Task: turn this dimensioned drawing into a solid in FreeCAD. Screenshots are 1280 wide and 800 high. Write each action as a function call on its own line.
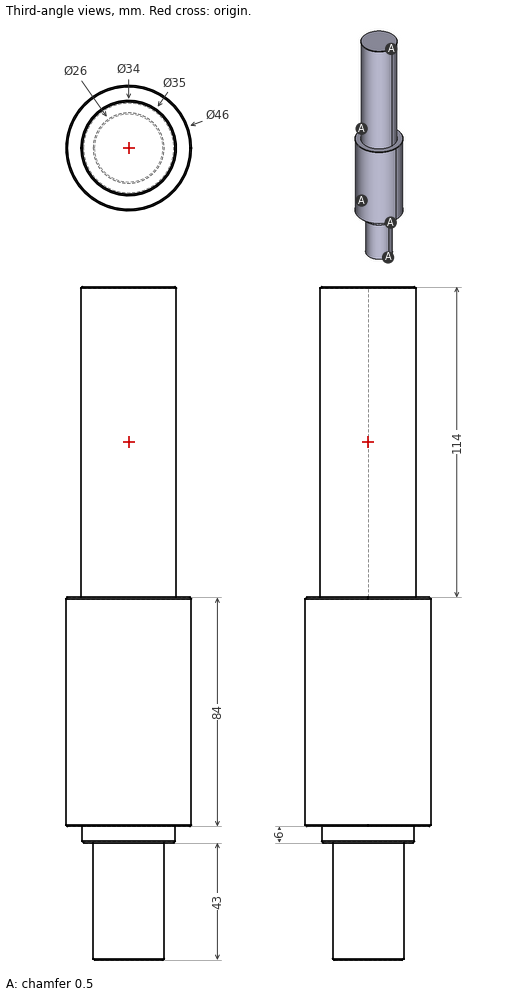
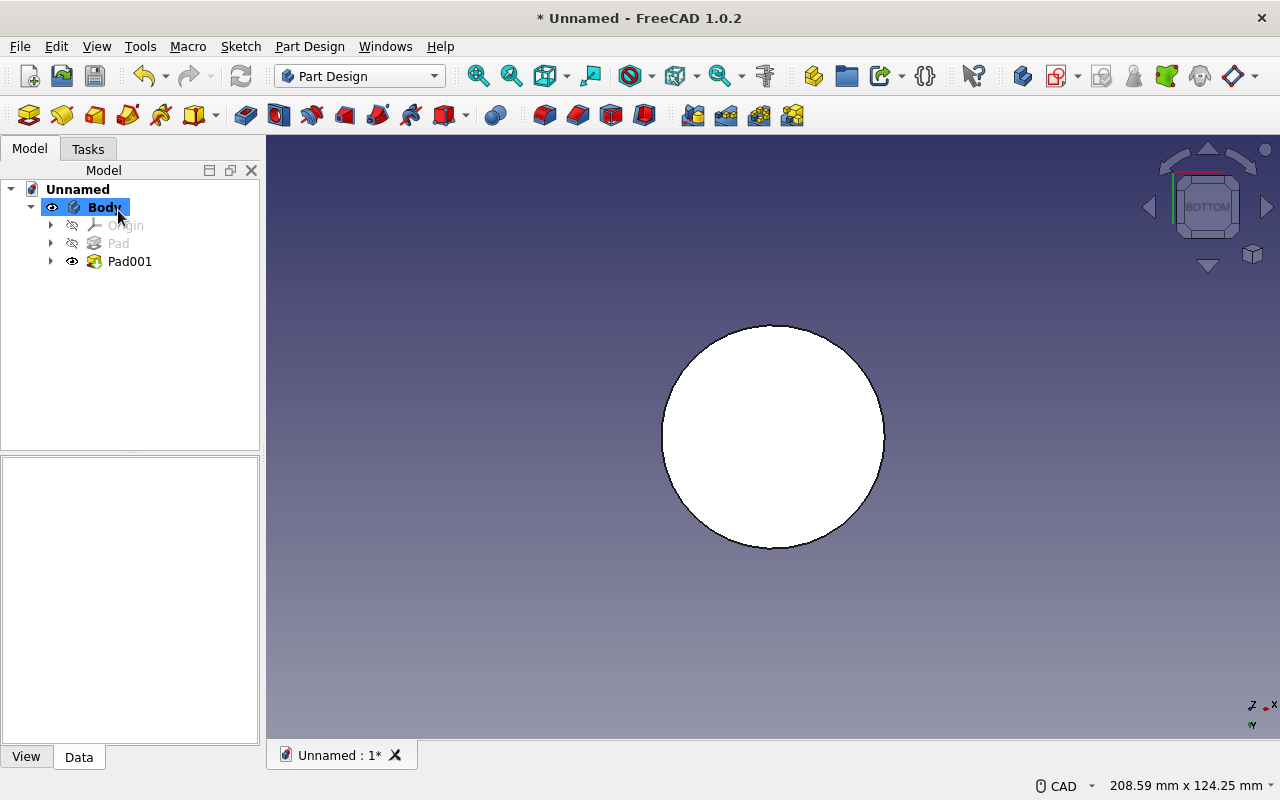
key(v)
key(f)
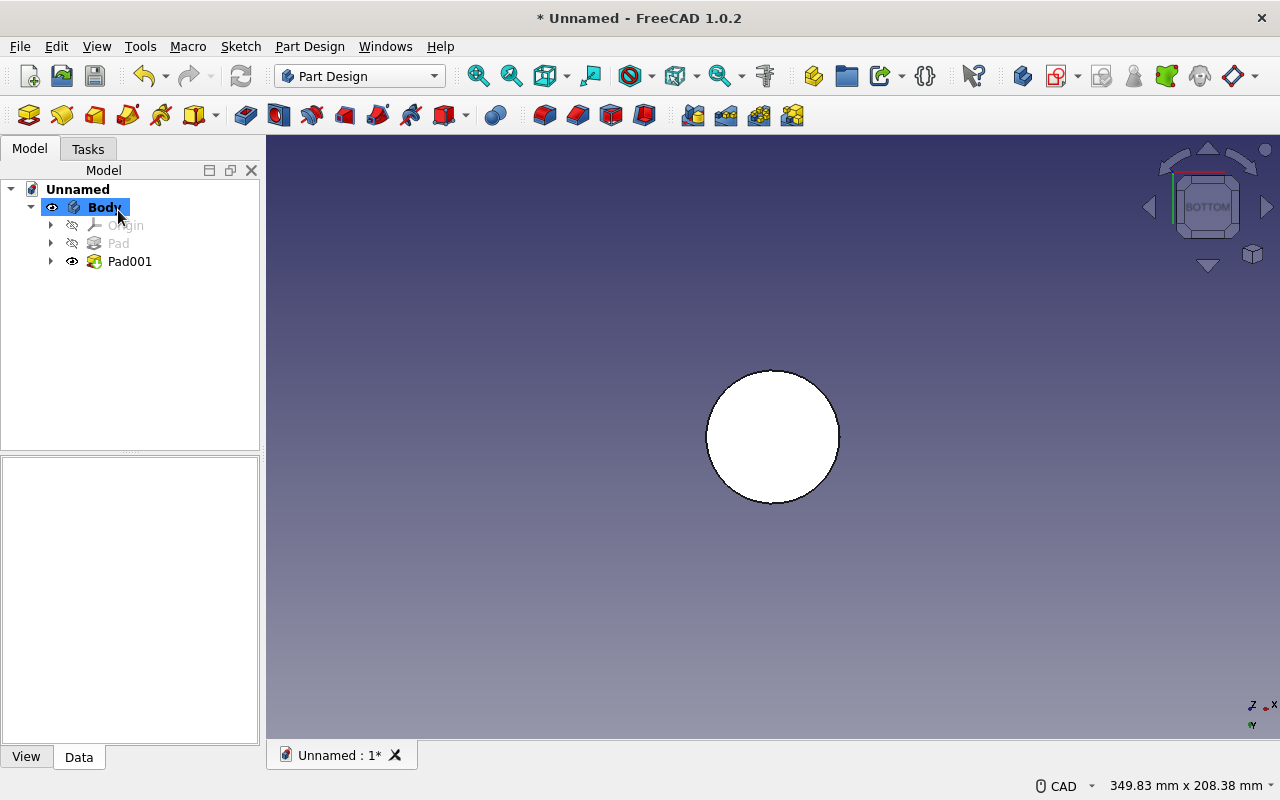
click(773, 436)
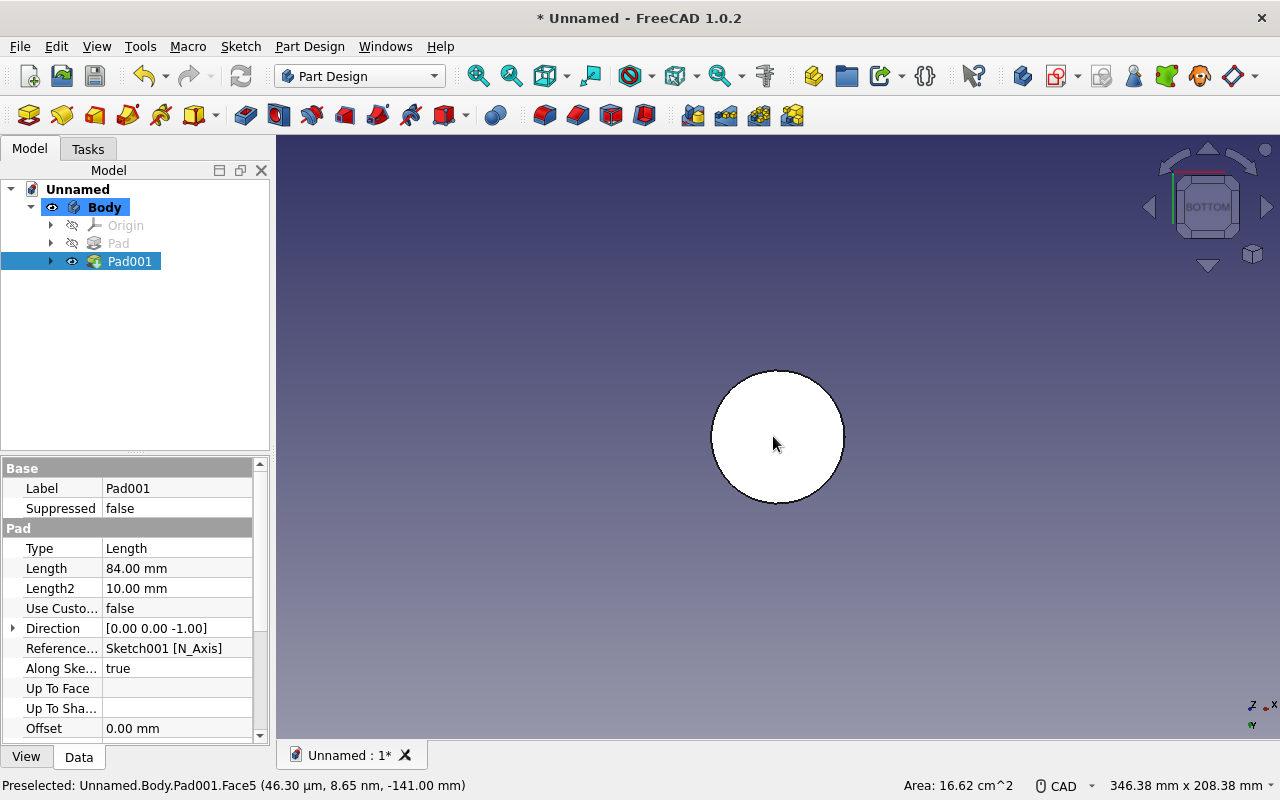
click(1056, 76)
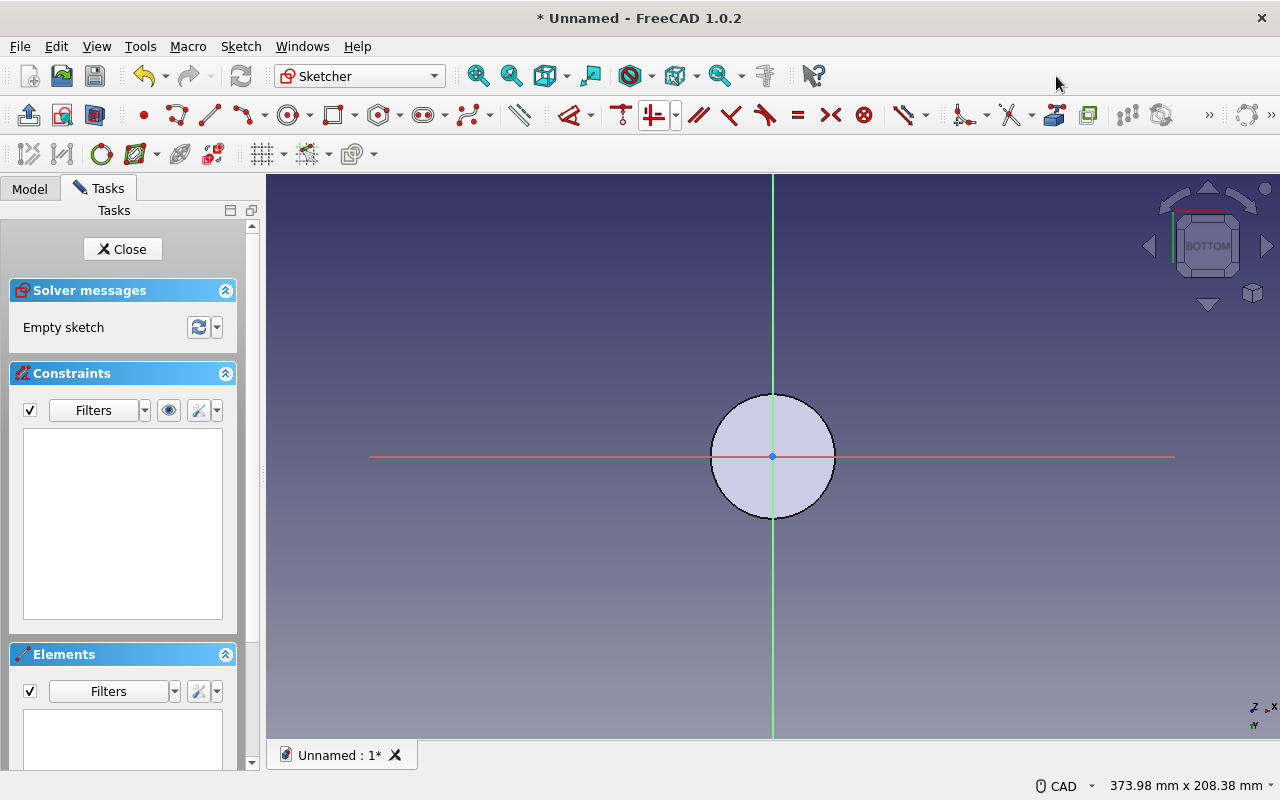
scroll(795, 456, up, 7)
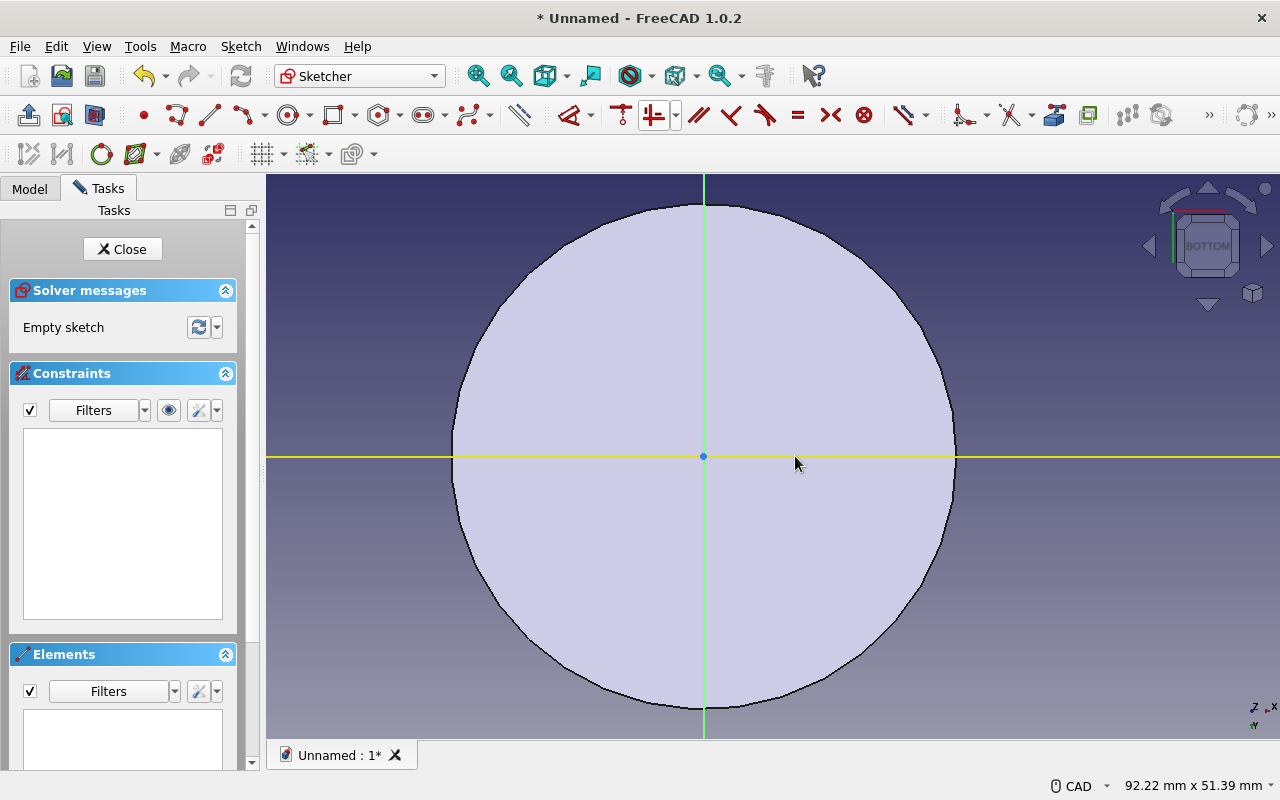
click(288, 116)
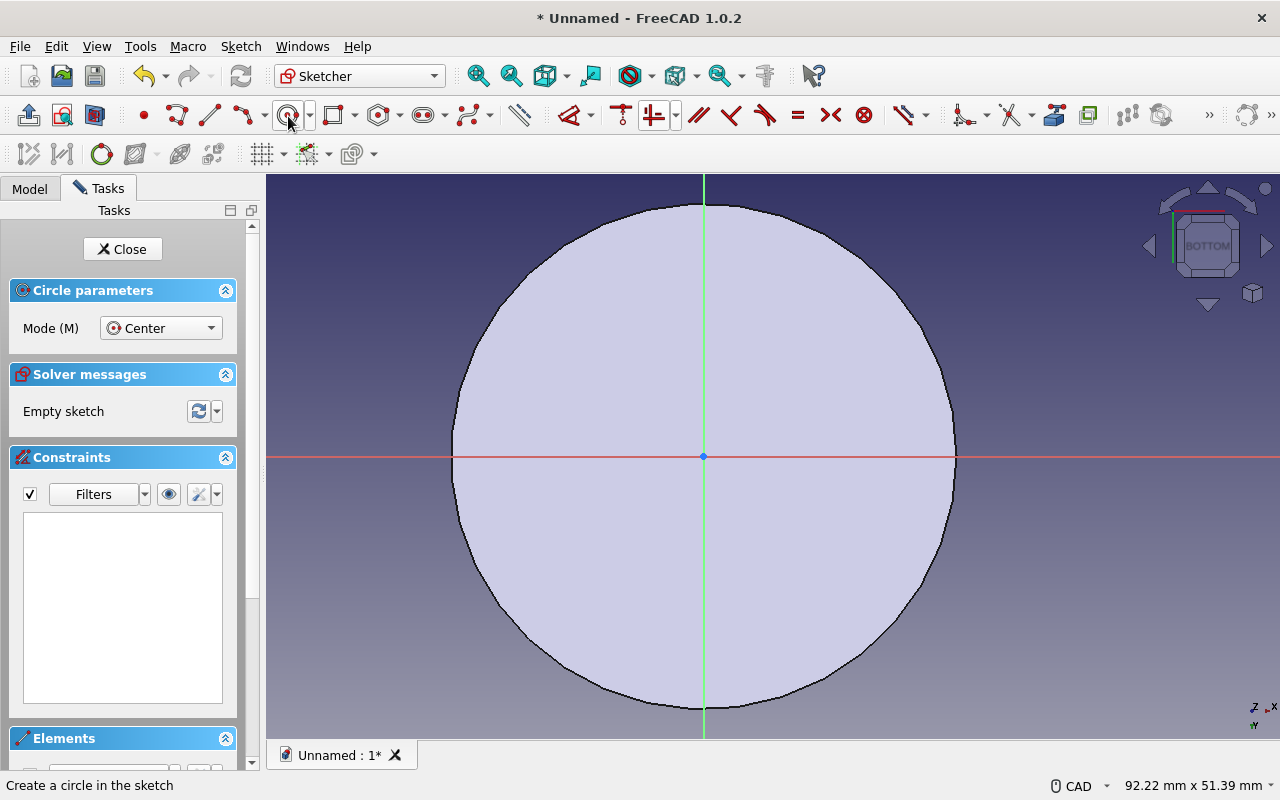
click(704, 456)
click(836, 324)
key(Escape)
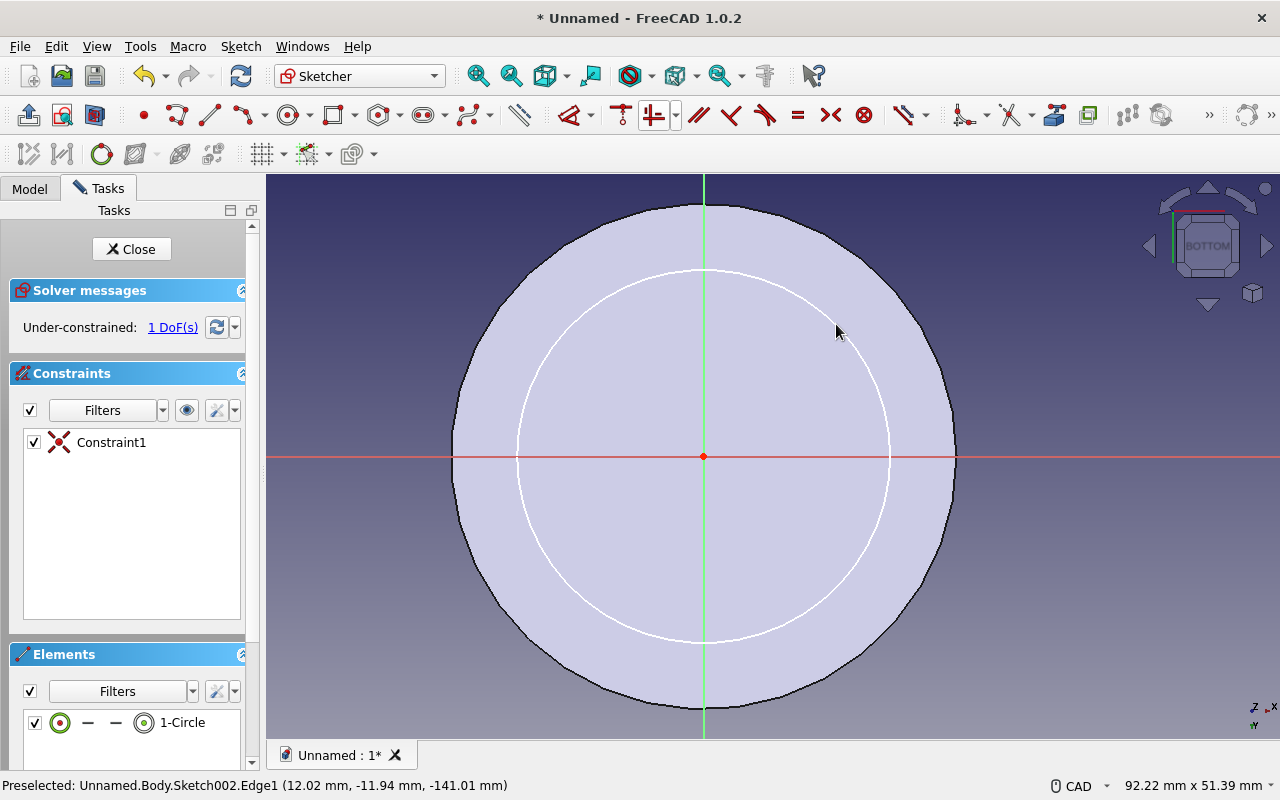
click(568, 116)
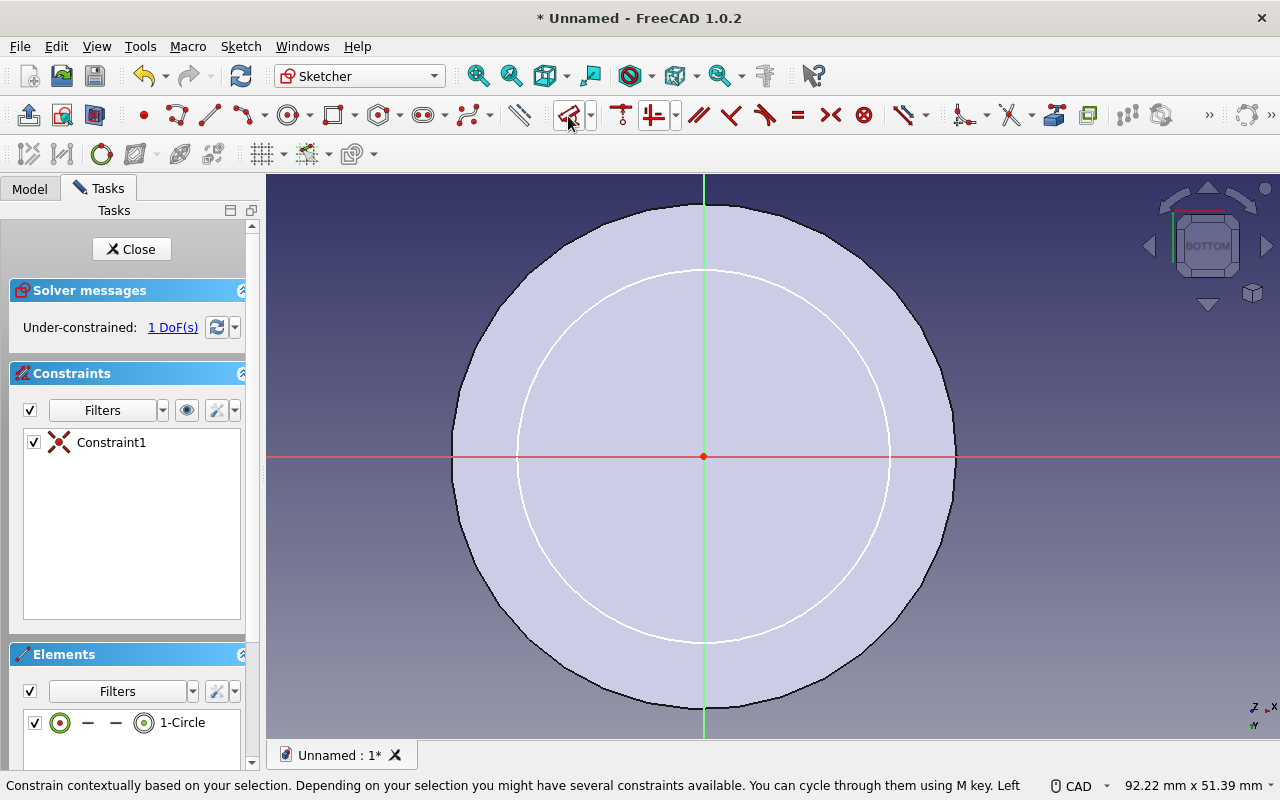
click(835, 324)
click(858, 301)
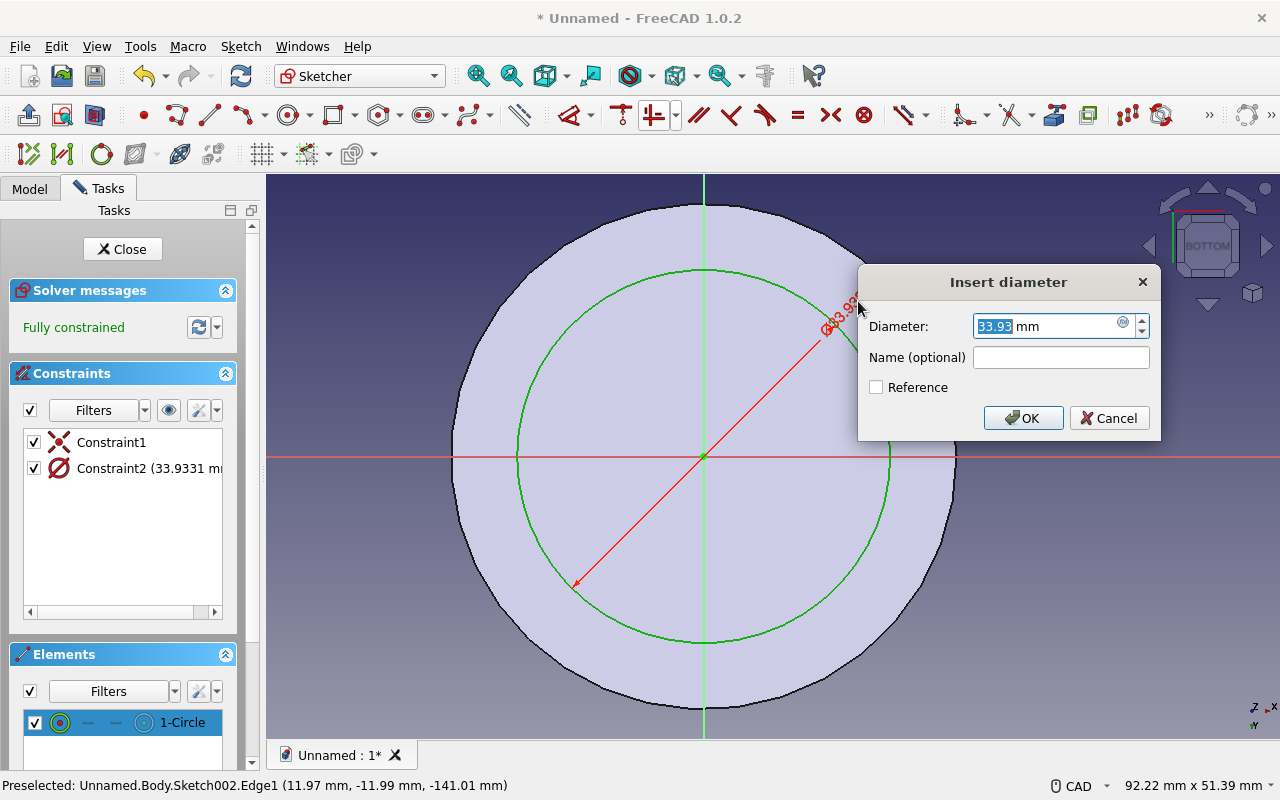
text(34)
key(Return)
key(Escape)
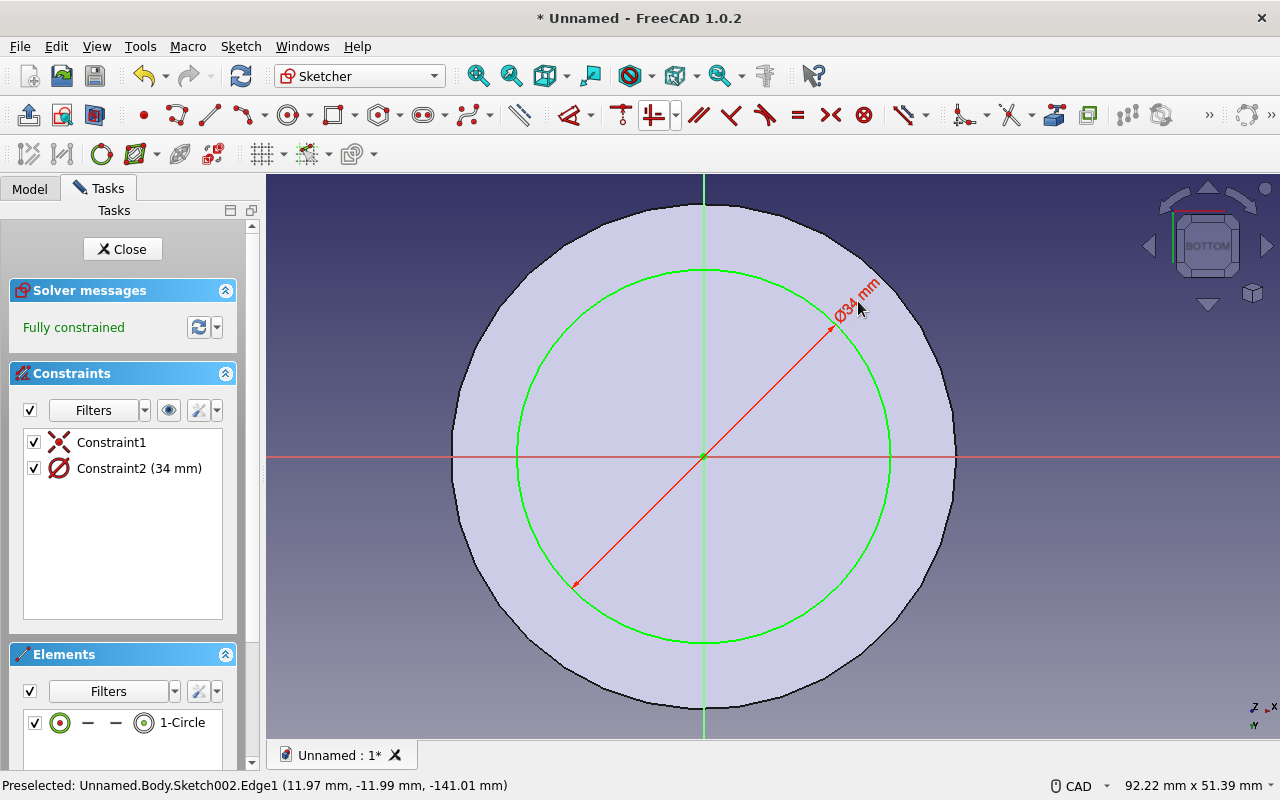
click(123, 249)